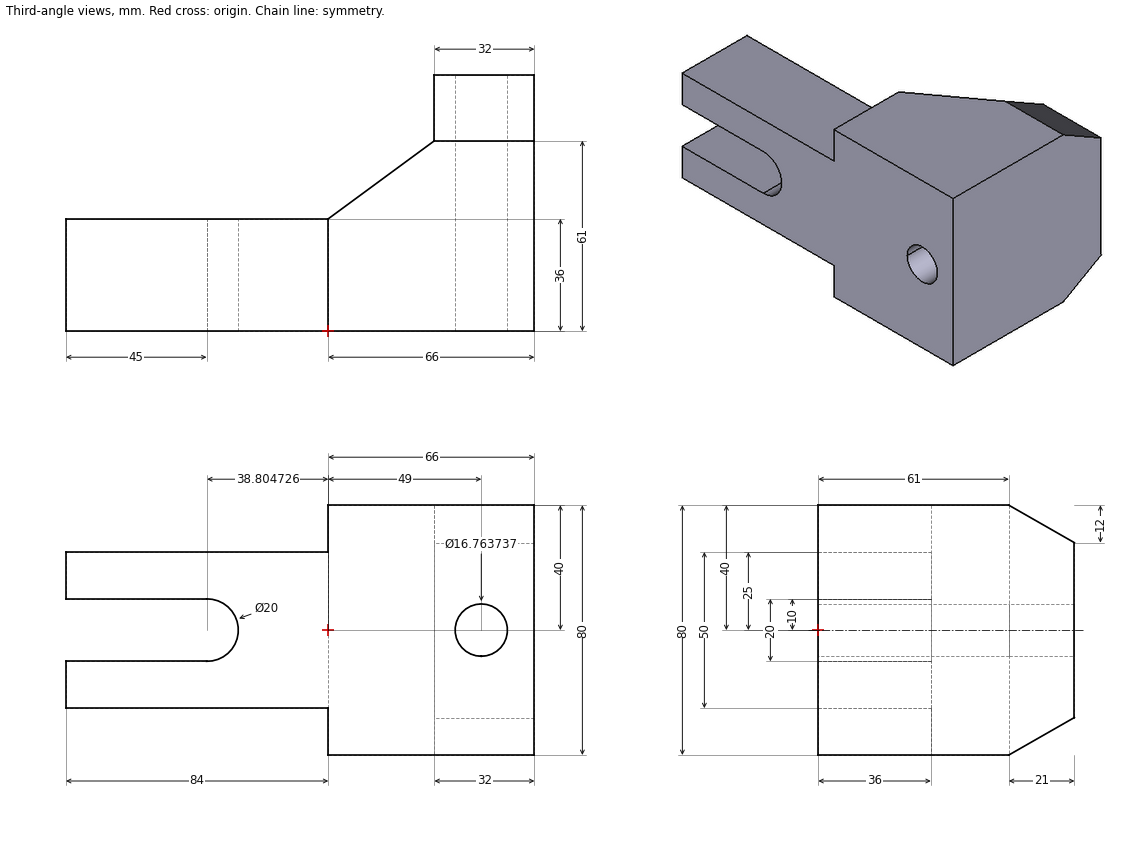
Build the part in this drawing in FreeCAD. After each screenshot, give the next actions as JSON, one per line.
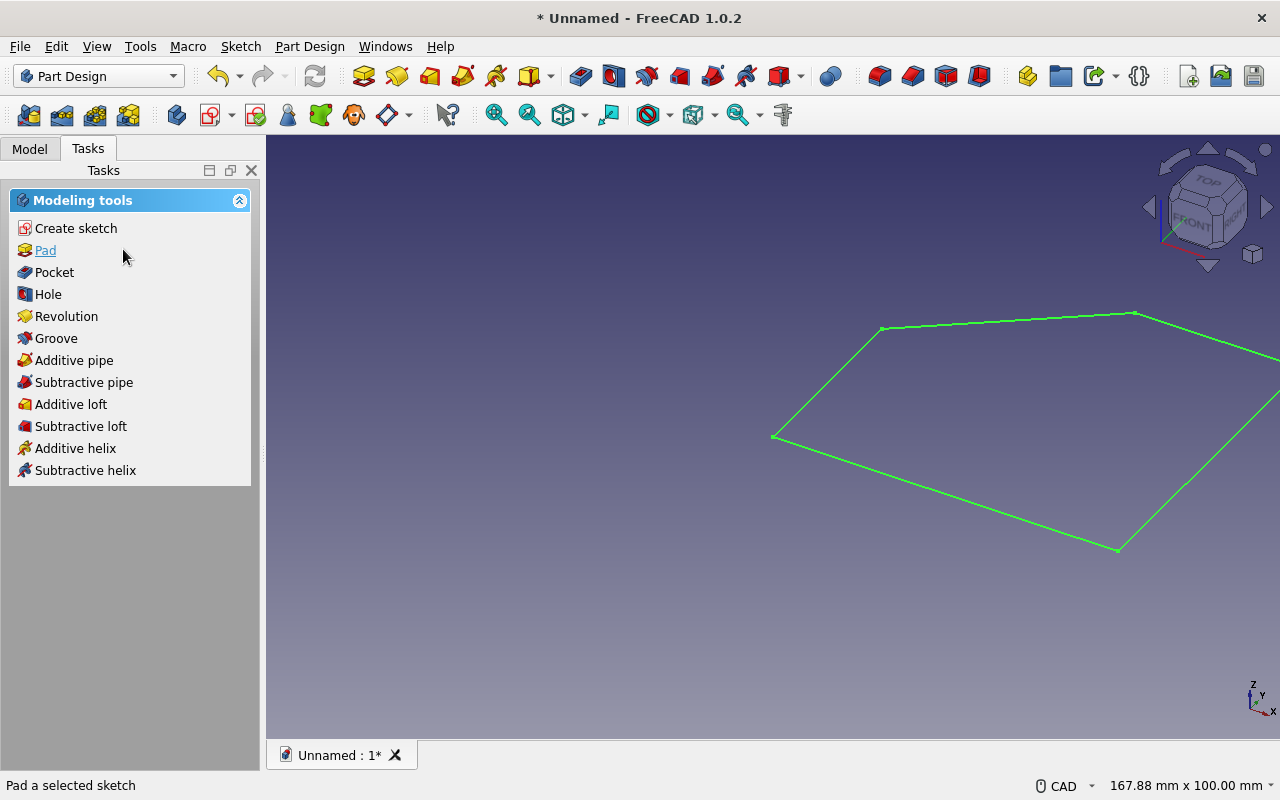
{"action": "left_click", "coordinate": [364, 76]}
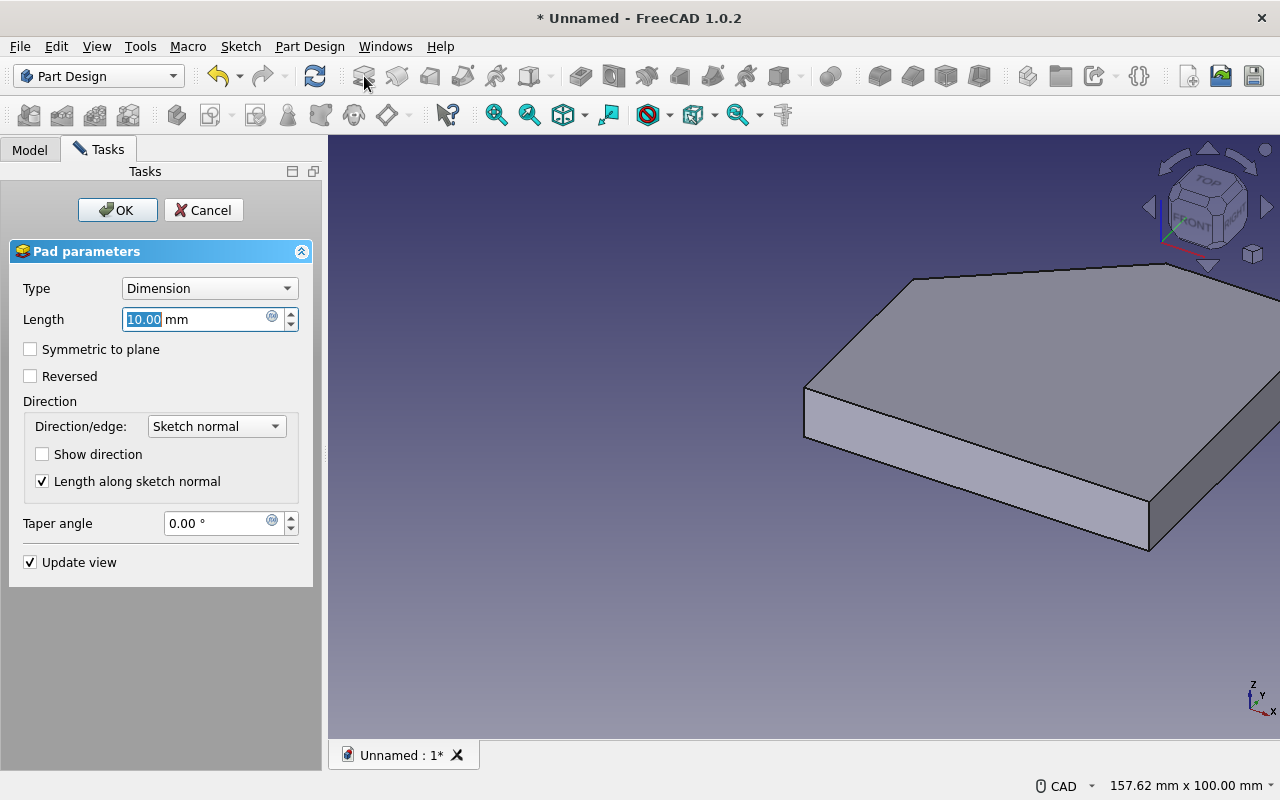
{"action": "type", "text": "80"}
{"action": "key", "text": "Tab"}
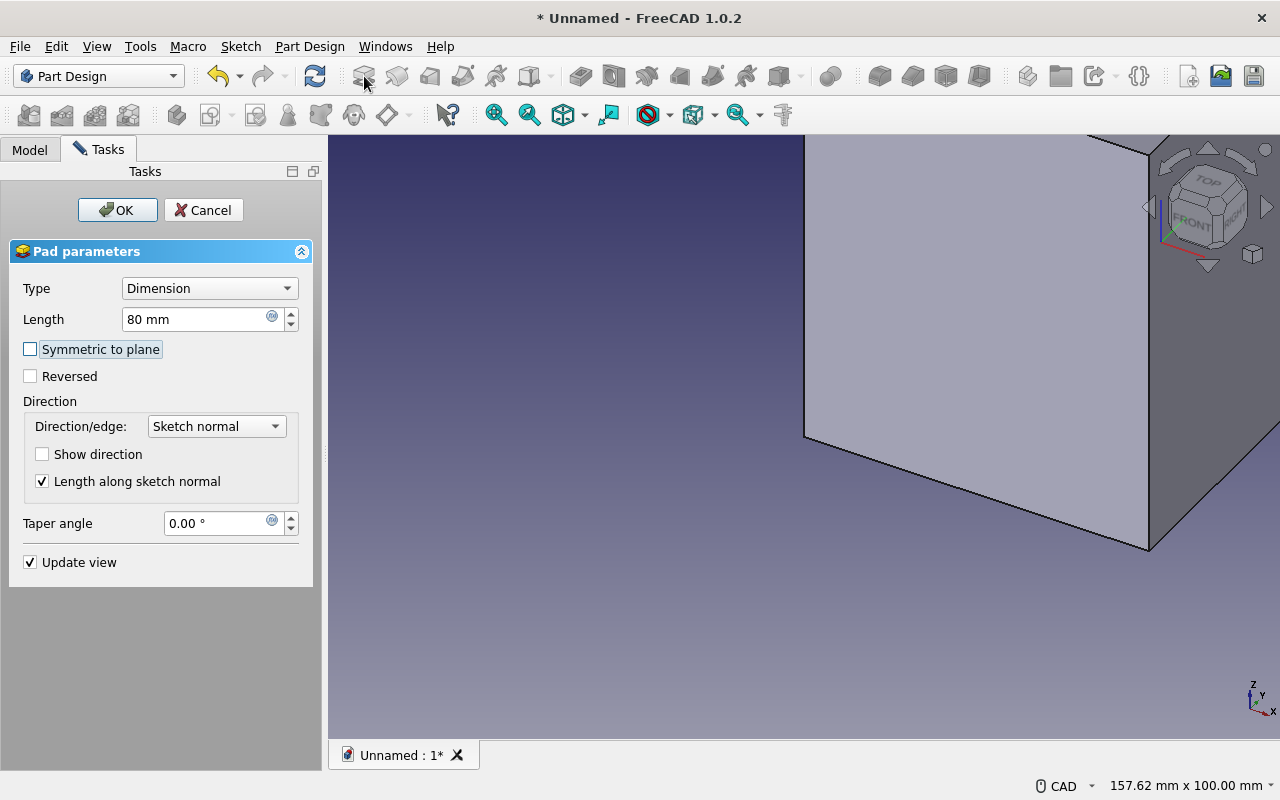
{"action": "left_click", "coordinate": [31, 349]}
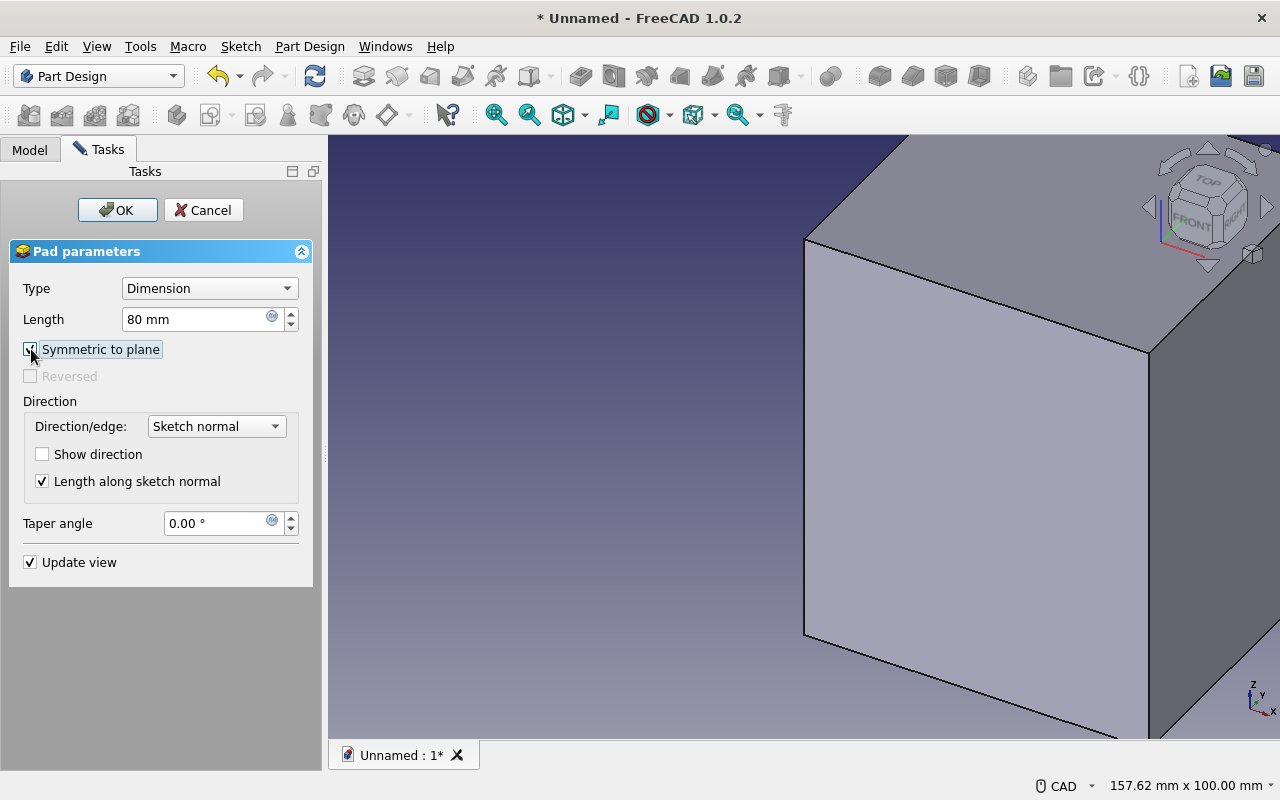
{"action": "left_click", "coordinate": [118, 210]}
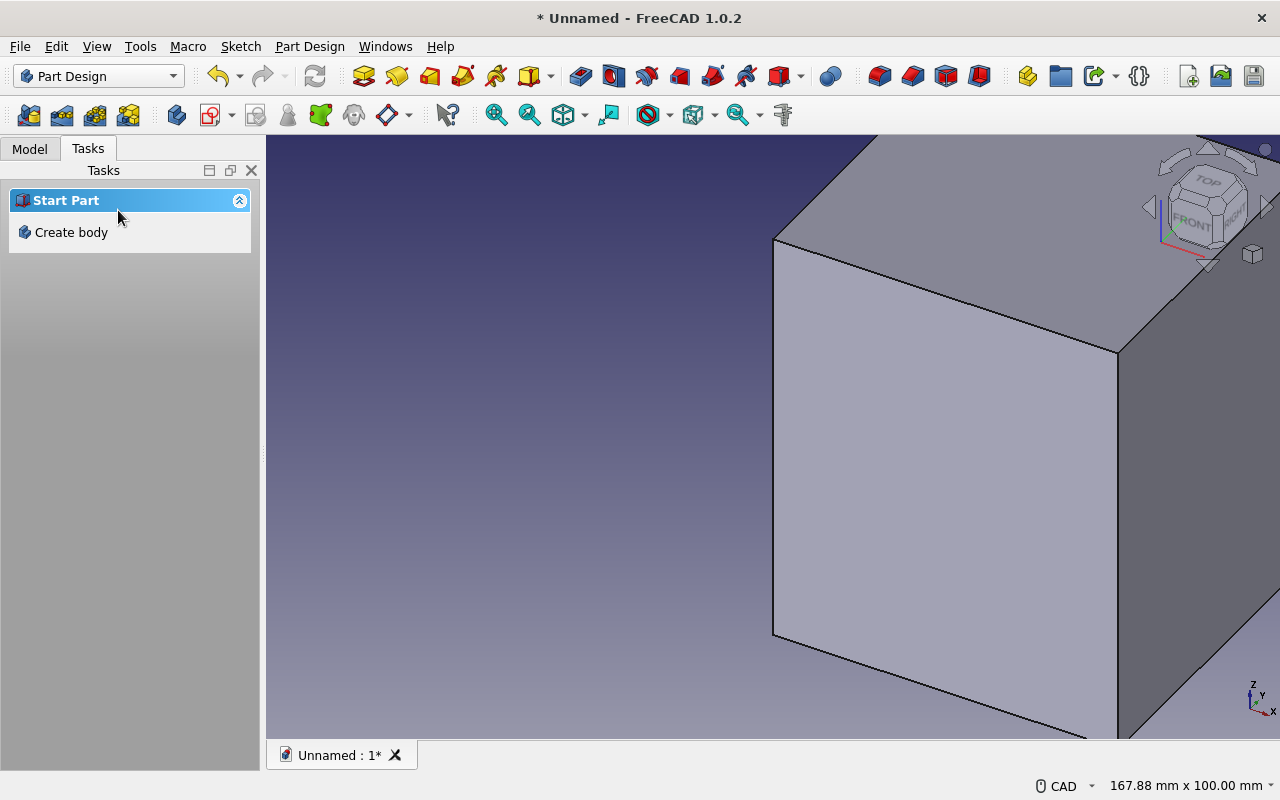
{"action": "left_click", "coordinate": [497, 116]}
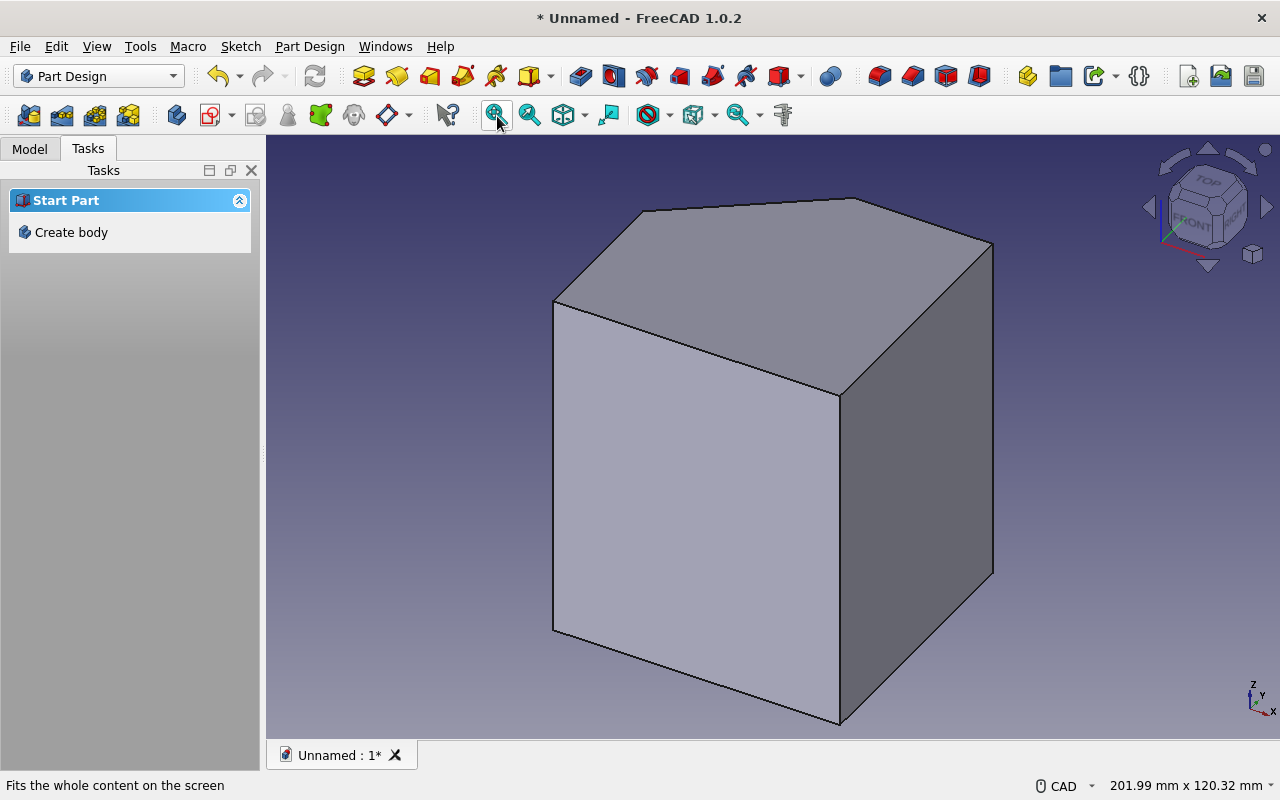
{"action": "key", "text": "4"}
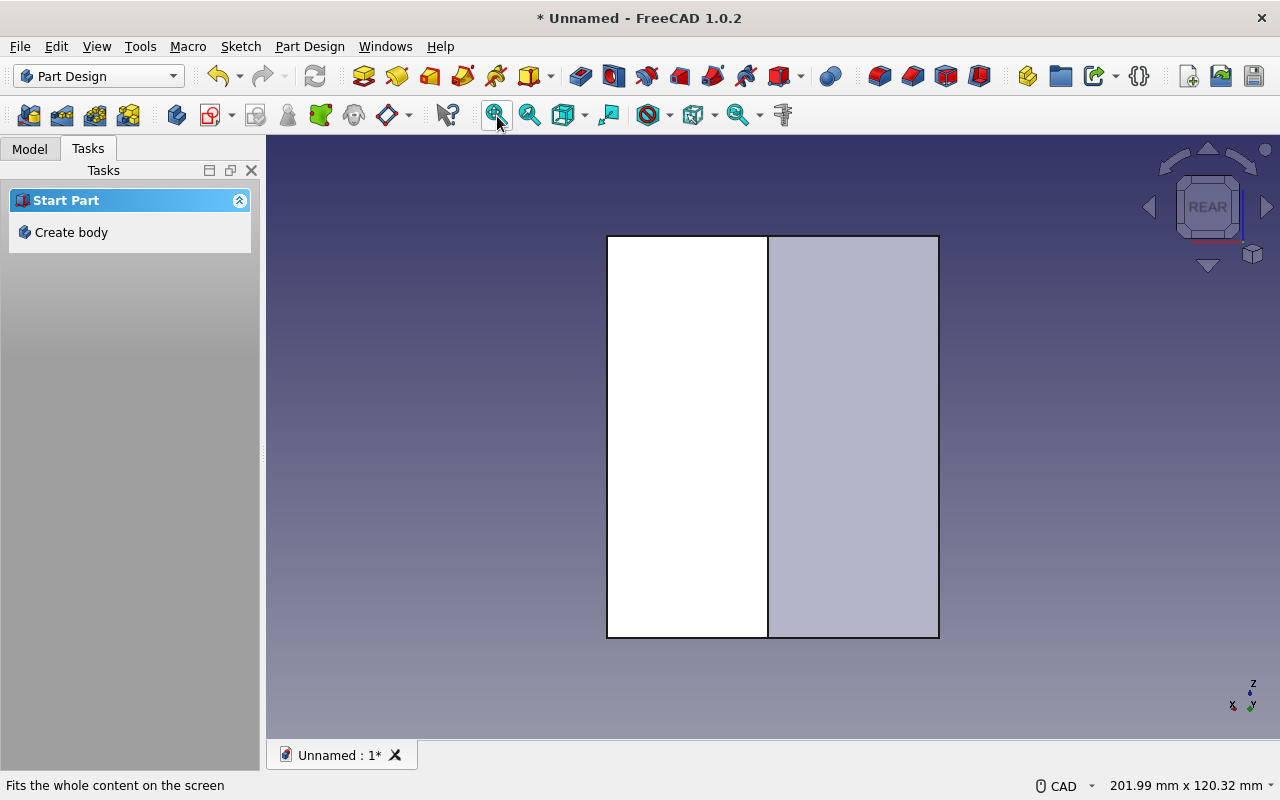
{"action": "left_click", "coordinate": [688, 321]}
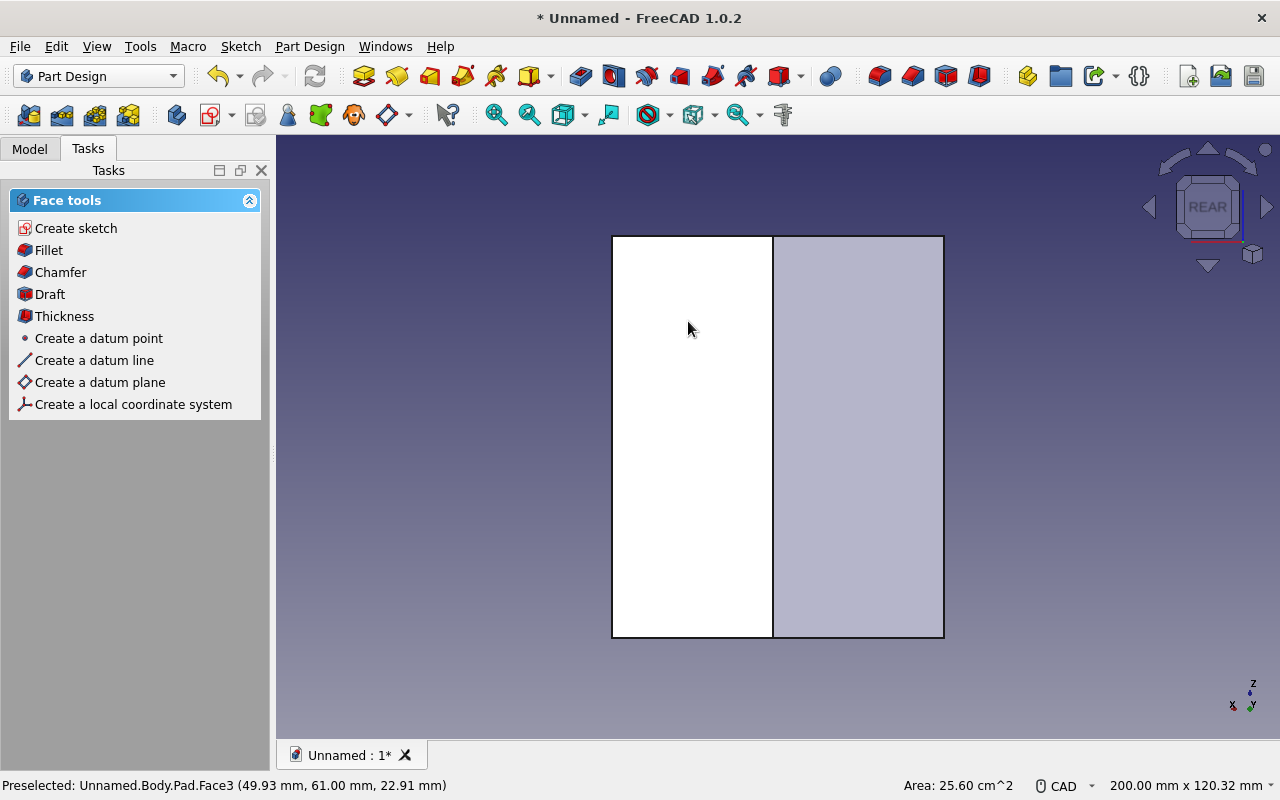
{"action": "left_click", "coordinate": [210, 116]}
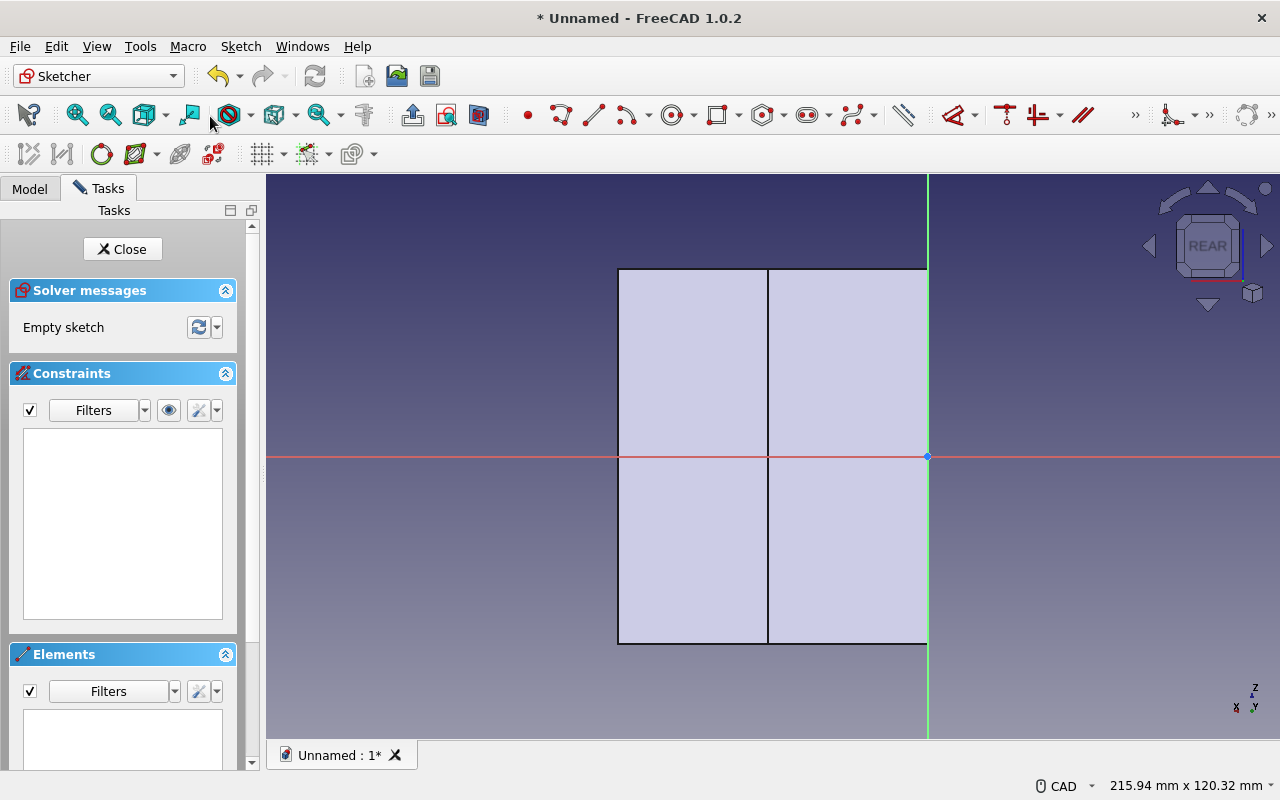
{"action": "key", "text": "g r"}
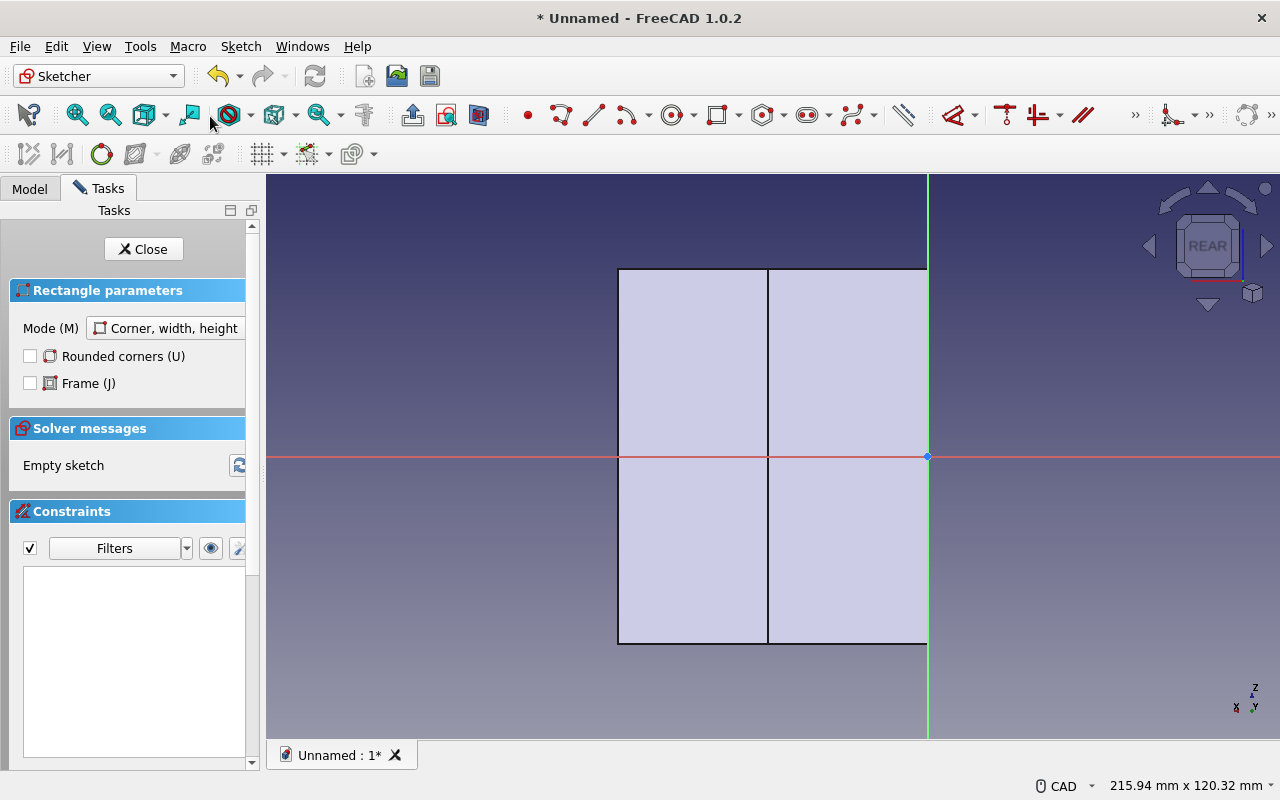
{"action": "left_click", "coordinate": [618, 269]}
{"action": "left_click", "coordinate": [768, 644]}